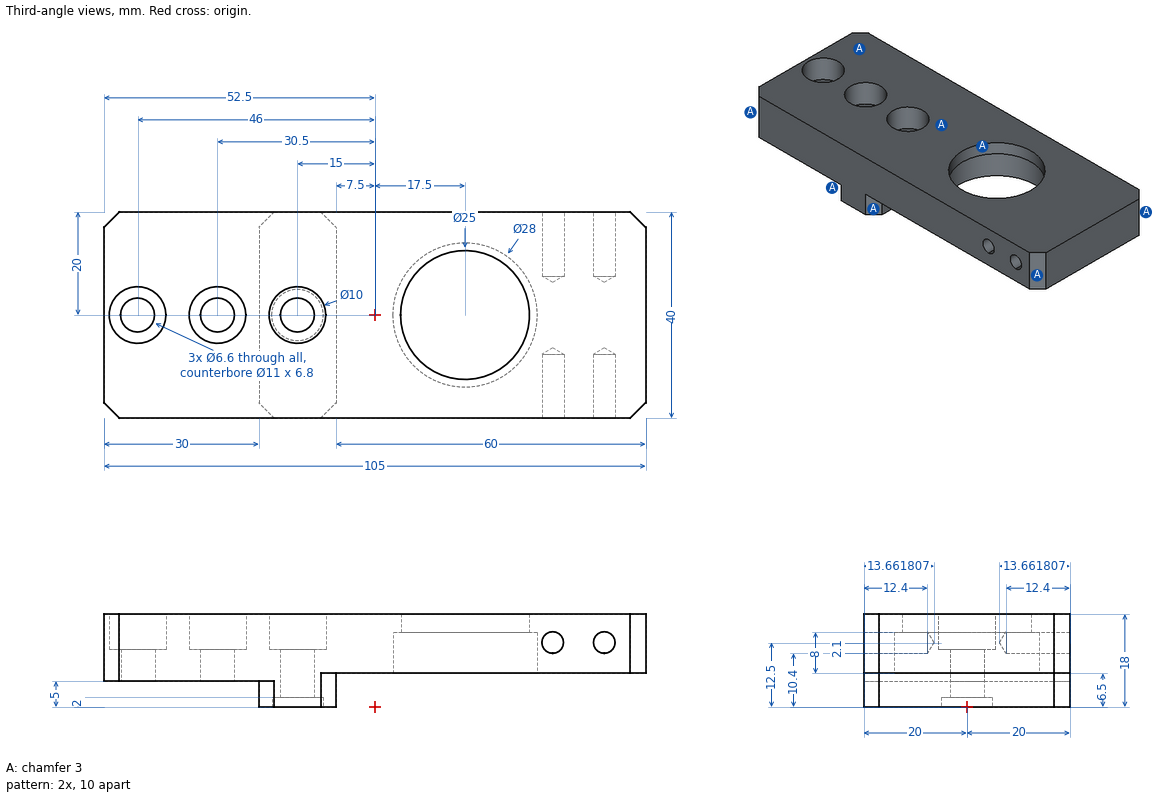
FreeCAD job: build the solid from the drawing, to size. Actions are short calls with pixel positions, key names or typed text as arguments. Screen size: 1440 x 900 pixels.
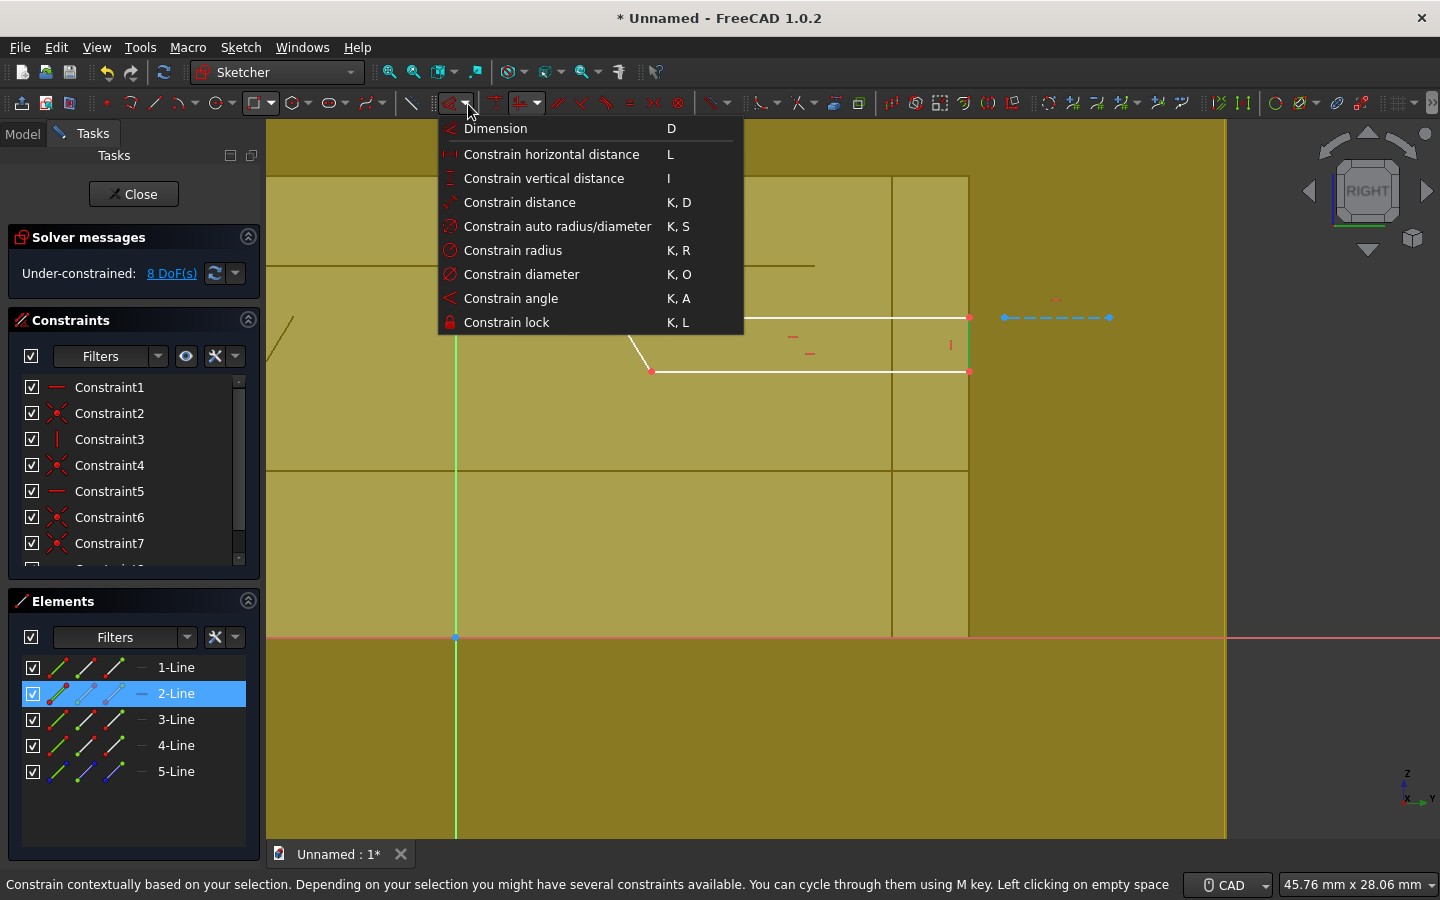
click(591, 178)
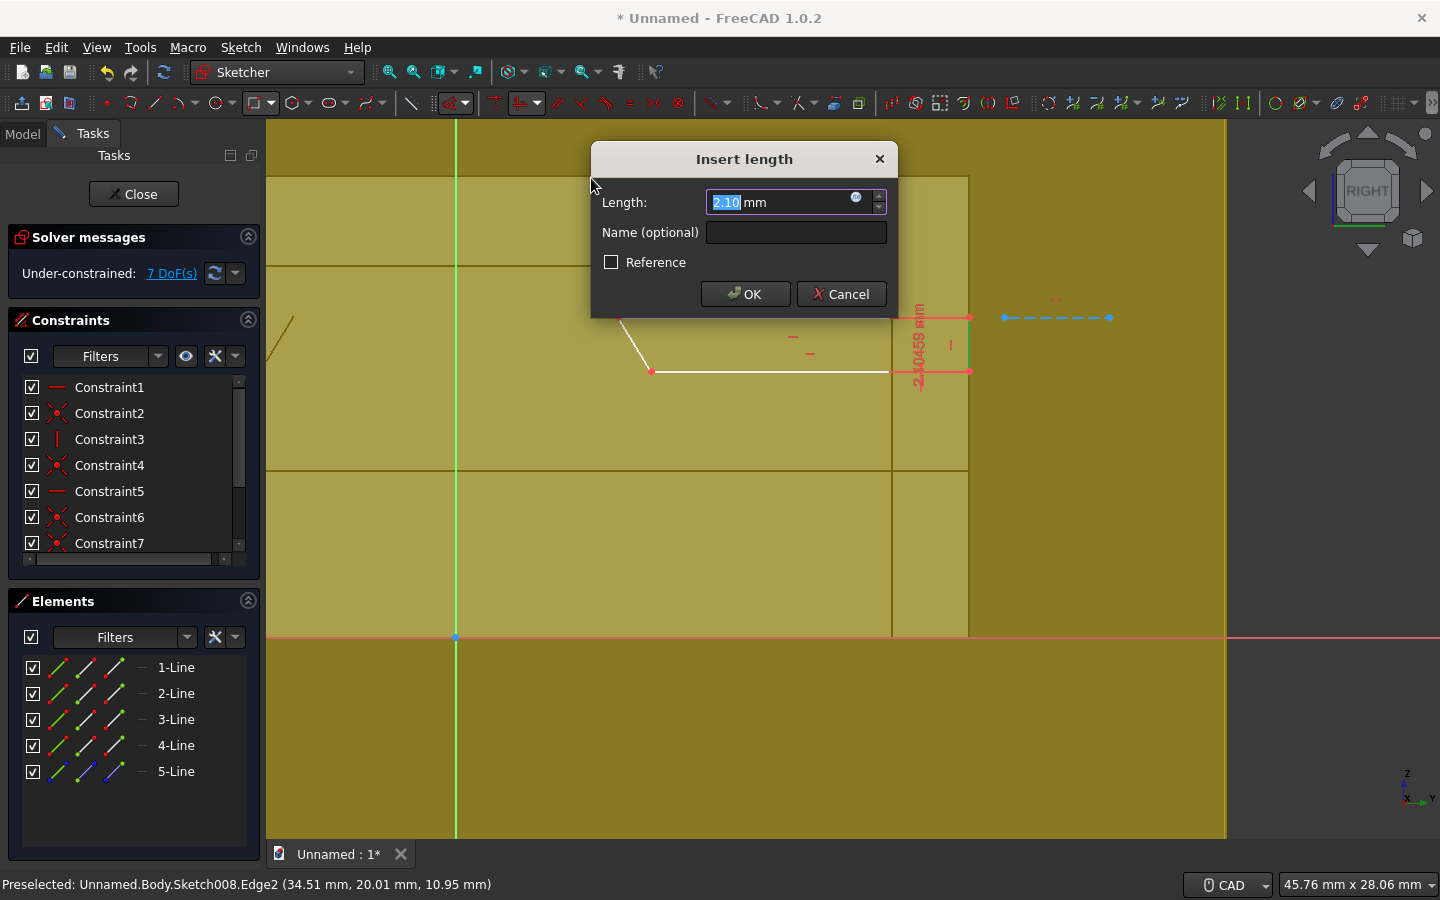
text(2.1)
key(Return)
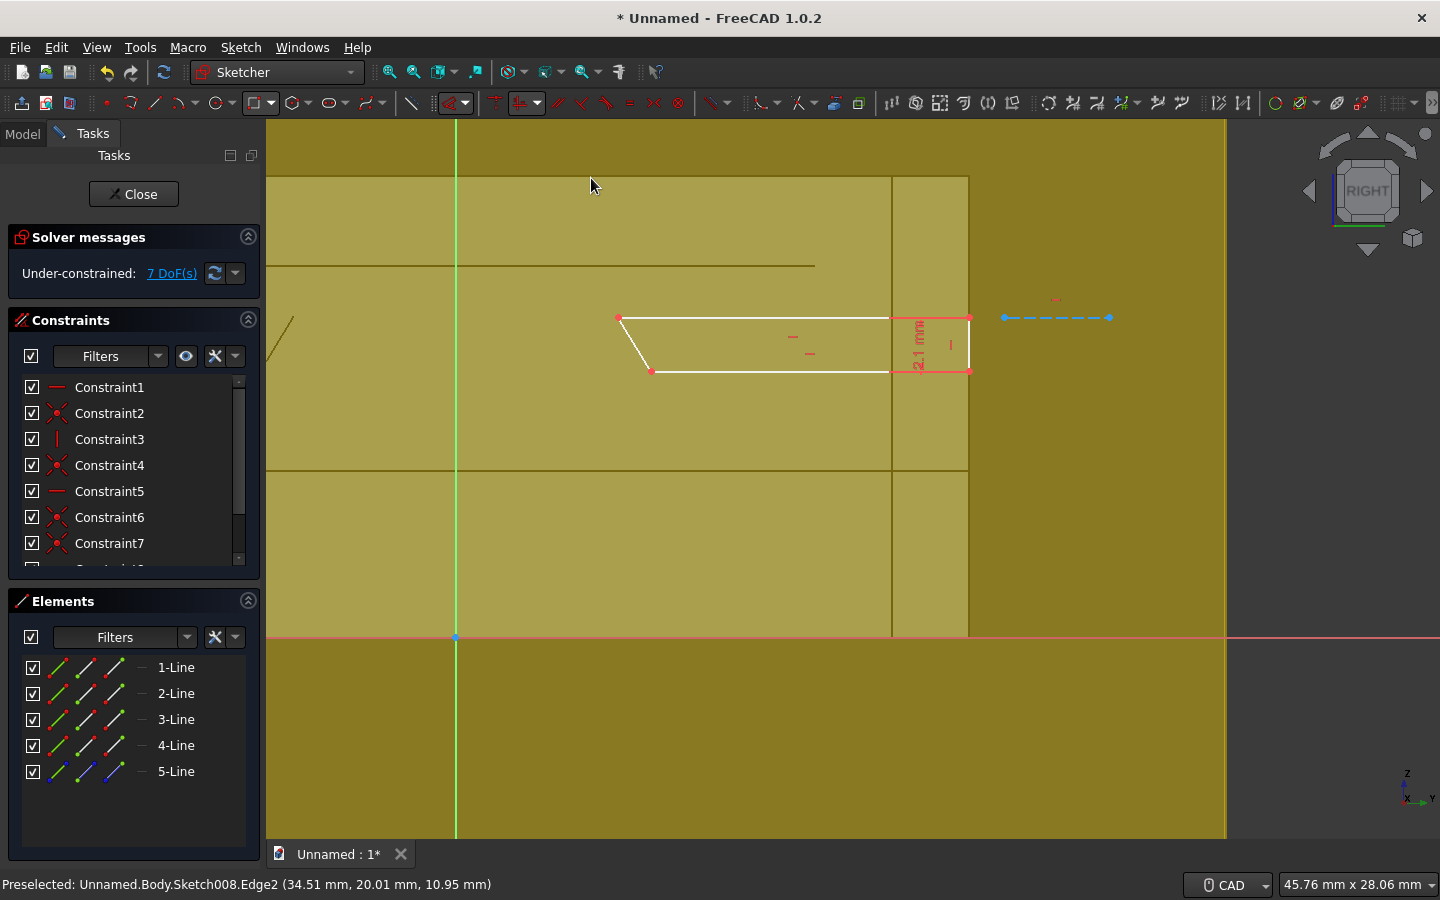
click(969, 372)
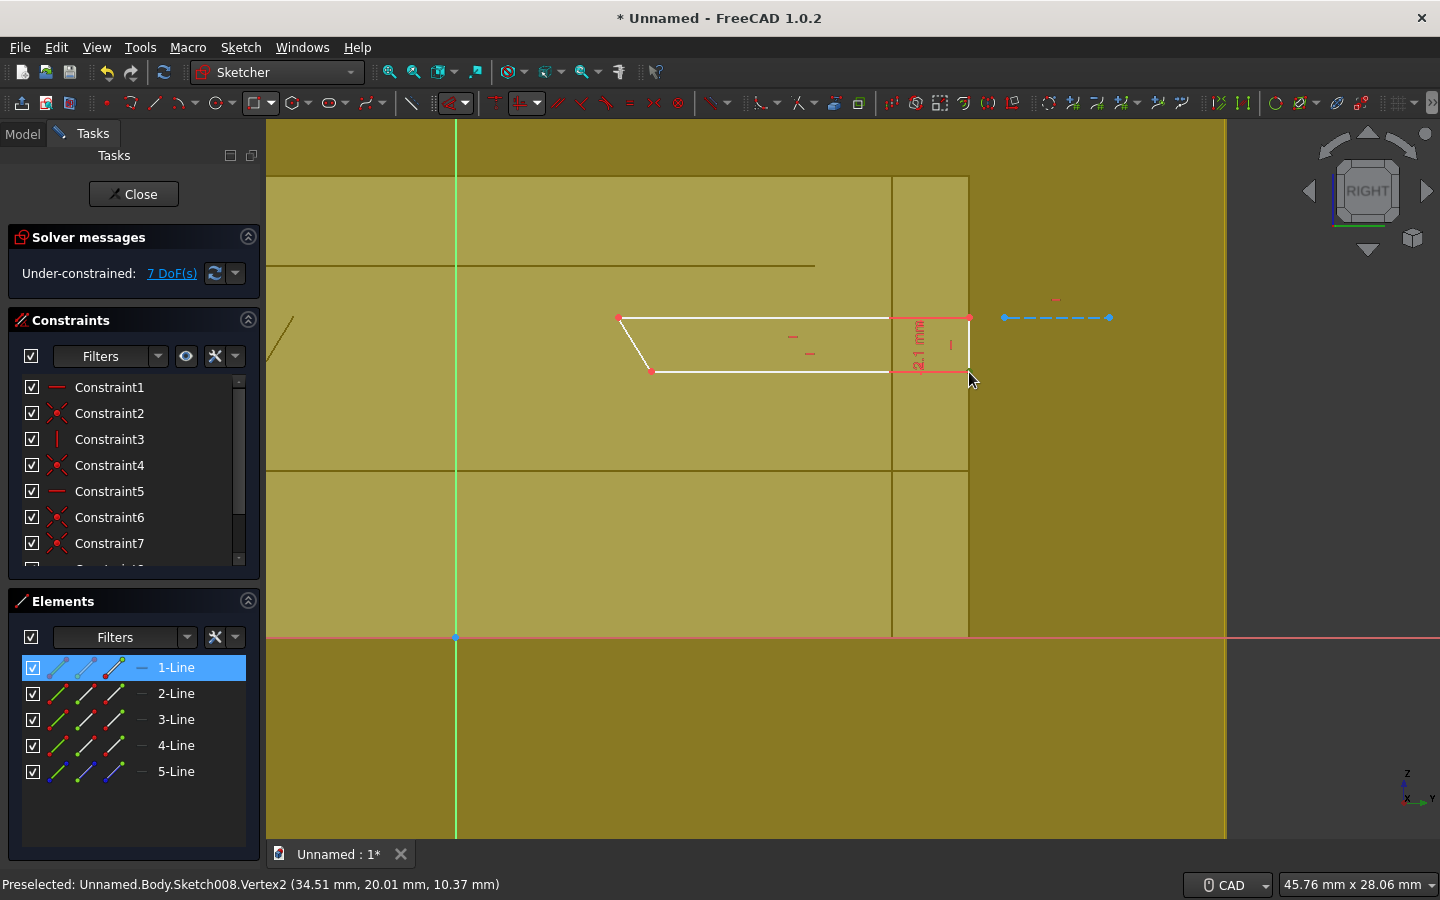
click(468, 104)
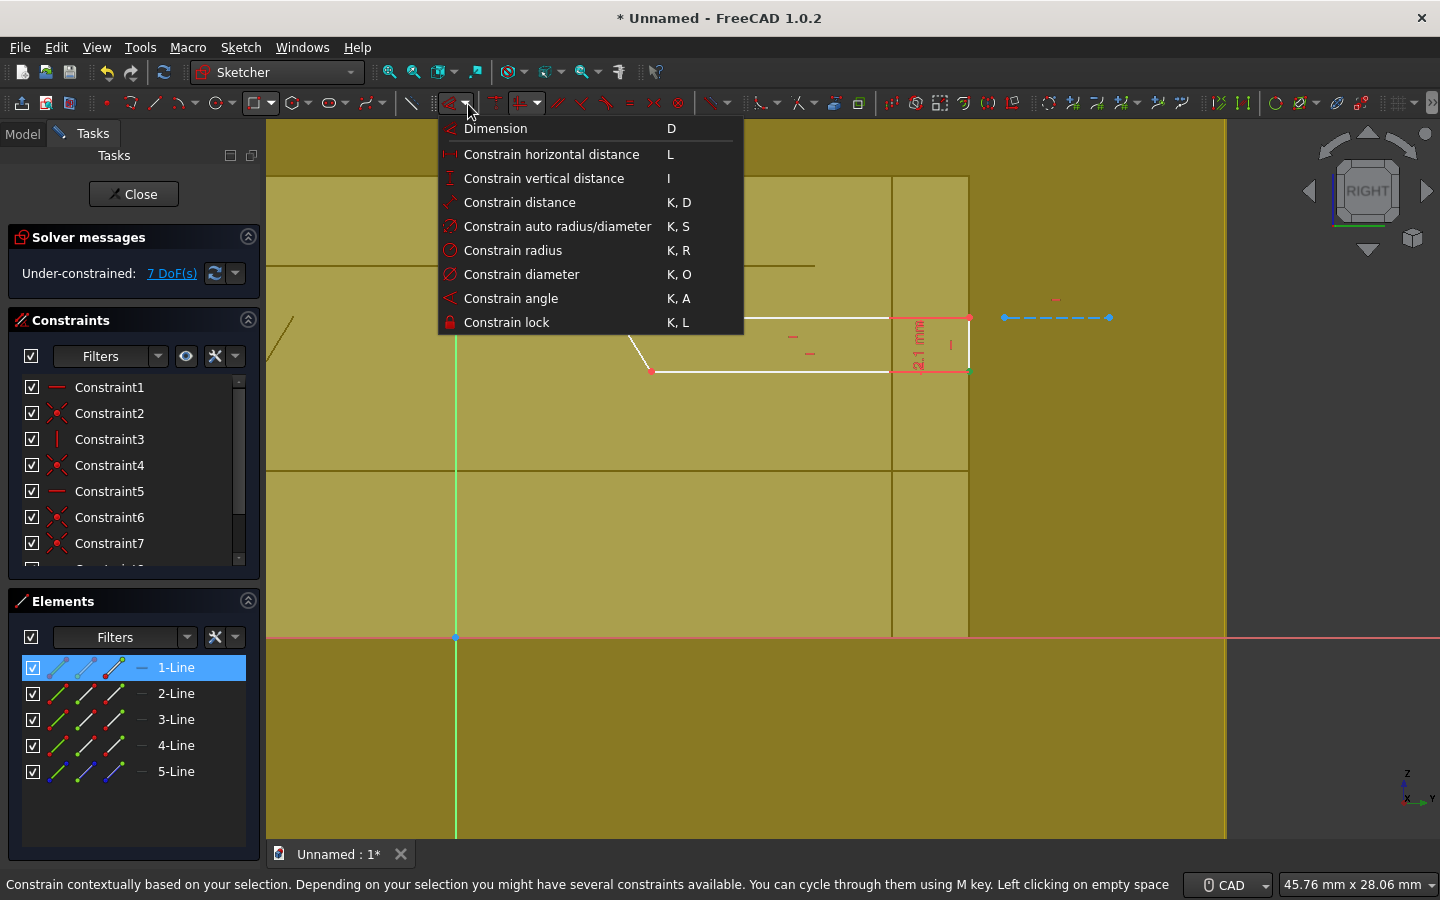
click(591, 154)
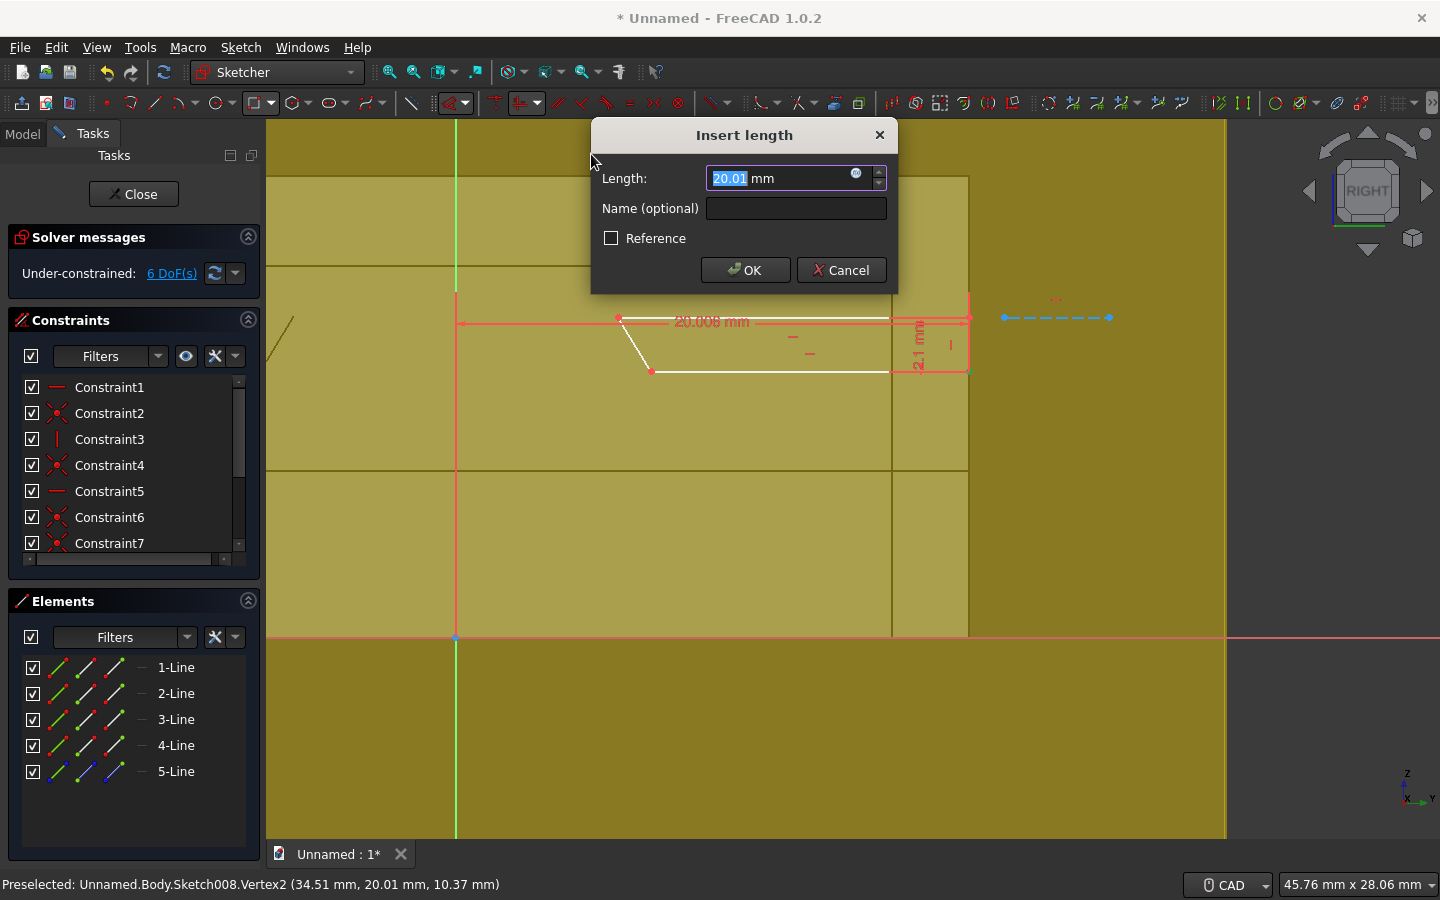
text(20)
key(Return)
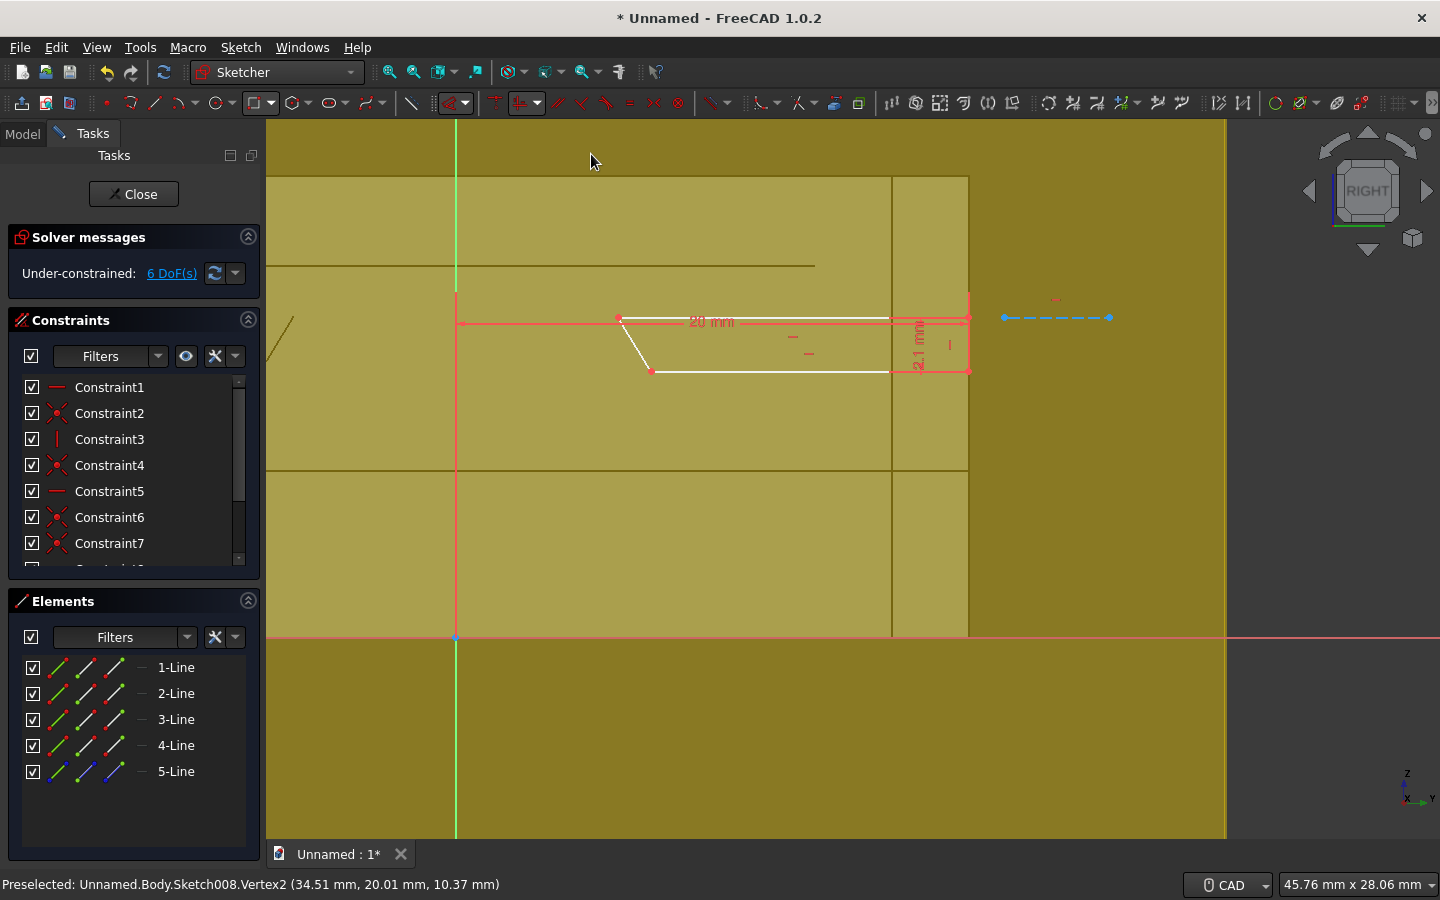
click(746, 372)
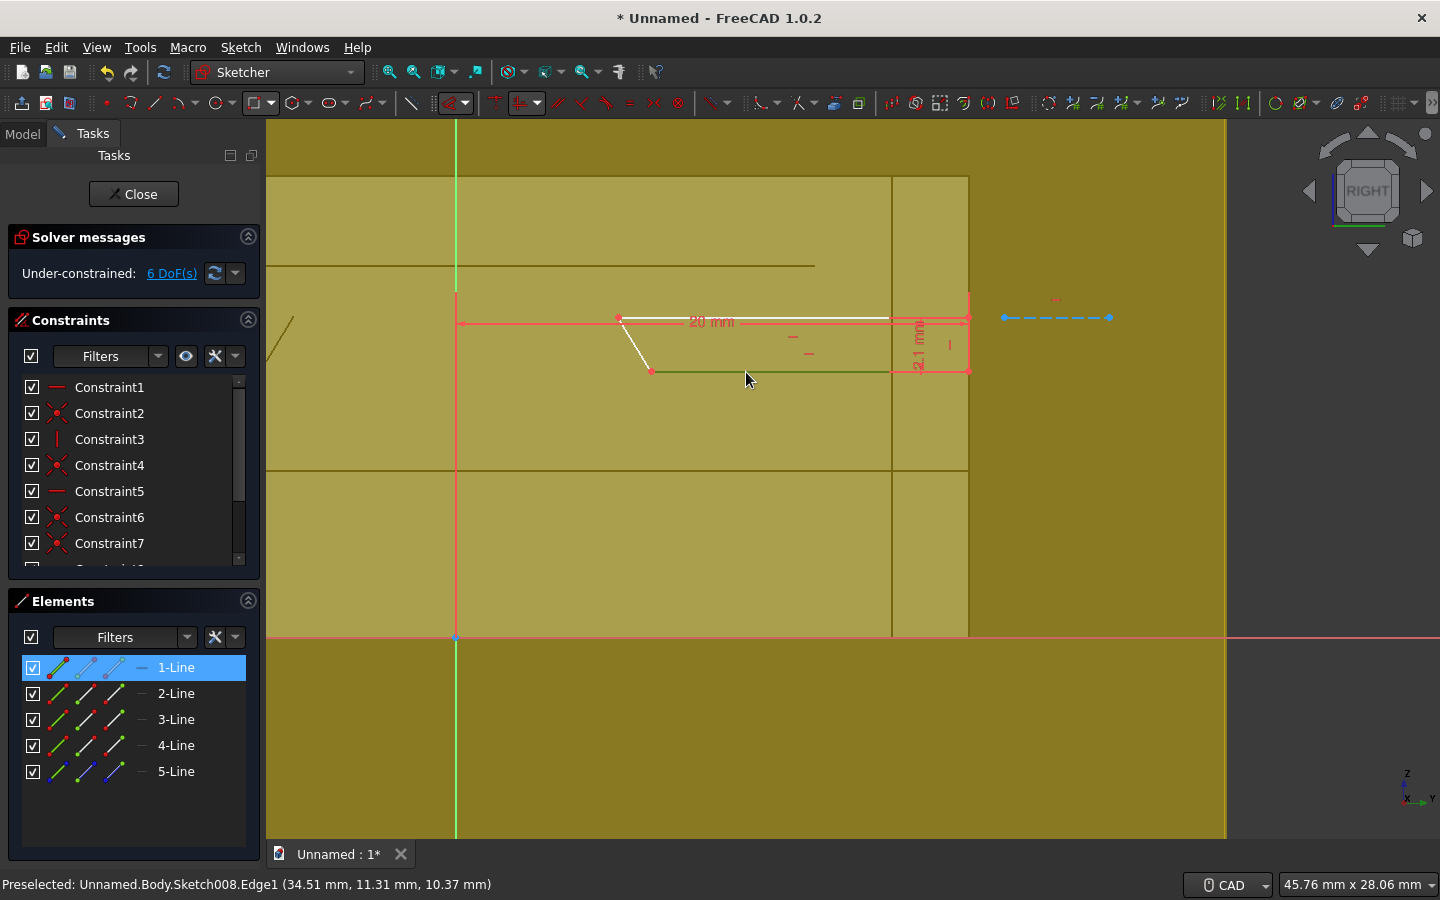
key(l)